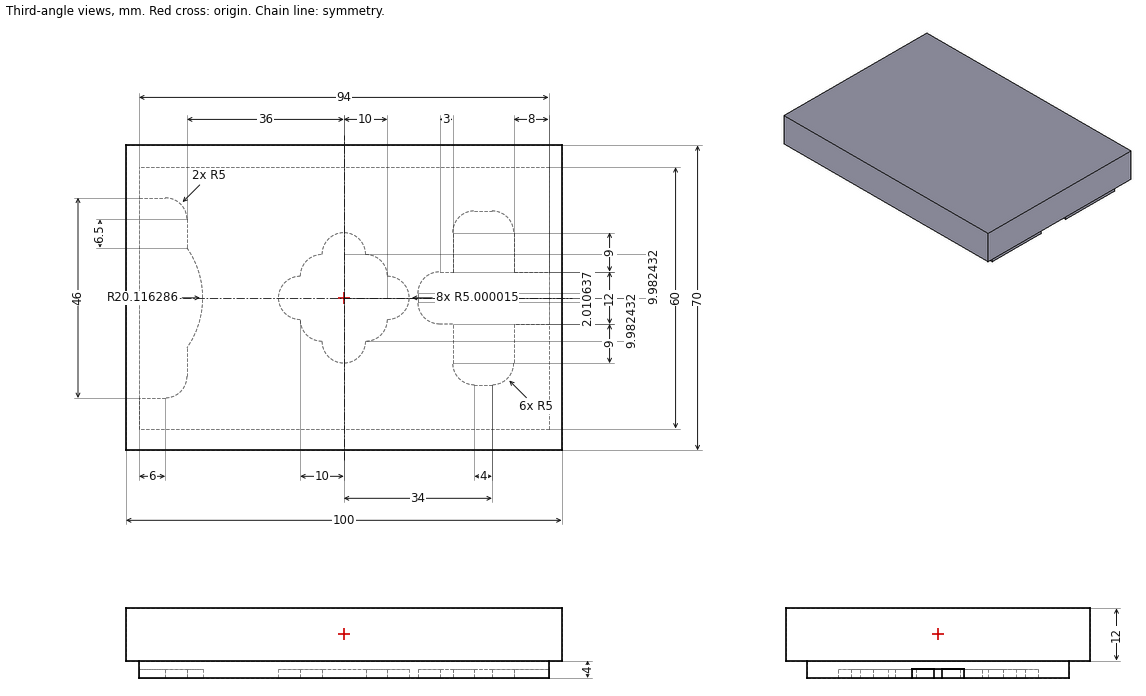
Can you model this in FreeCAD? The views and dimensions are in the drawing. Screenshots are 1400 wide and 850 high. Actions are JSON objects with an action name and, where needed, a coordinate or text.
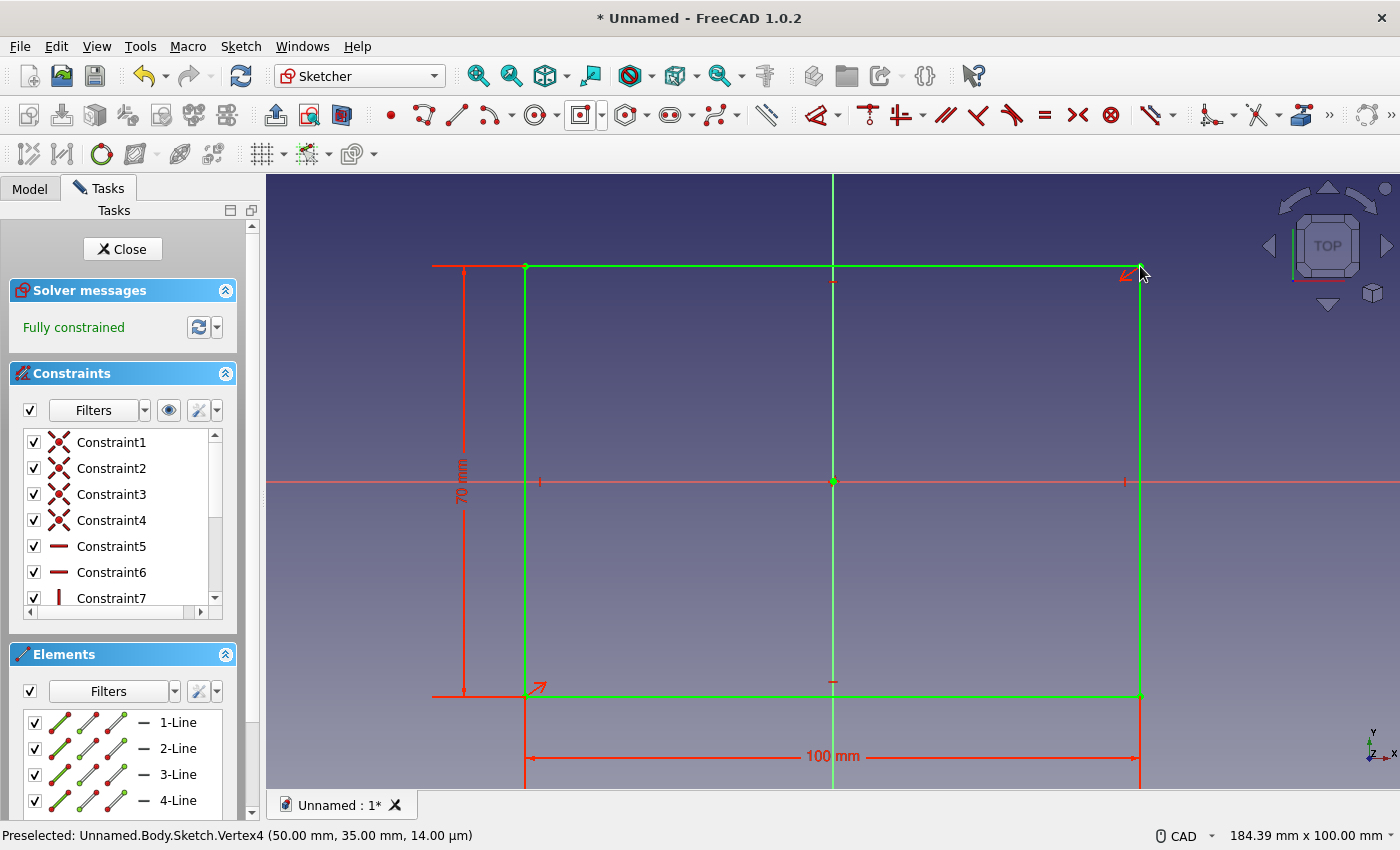
{"action": "left_click", "coordinate": [123, 249]}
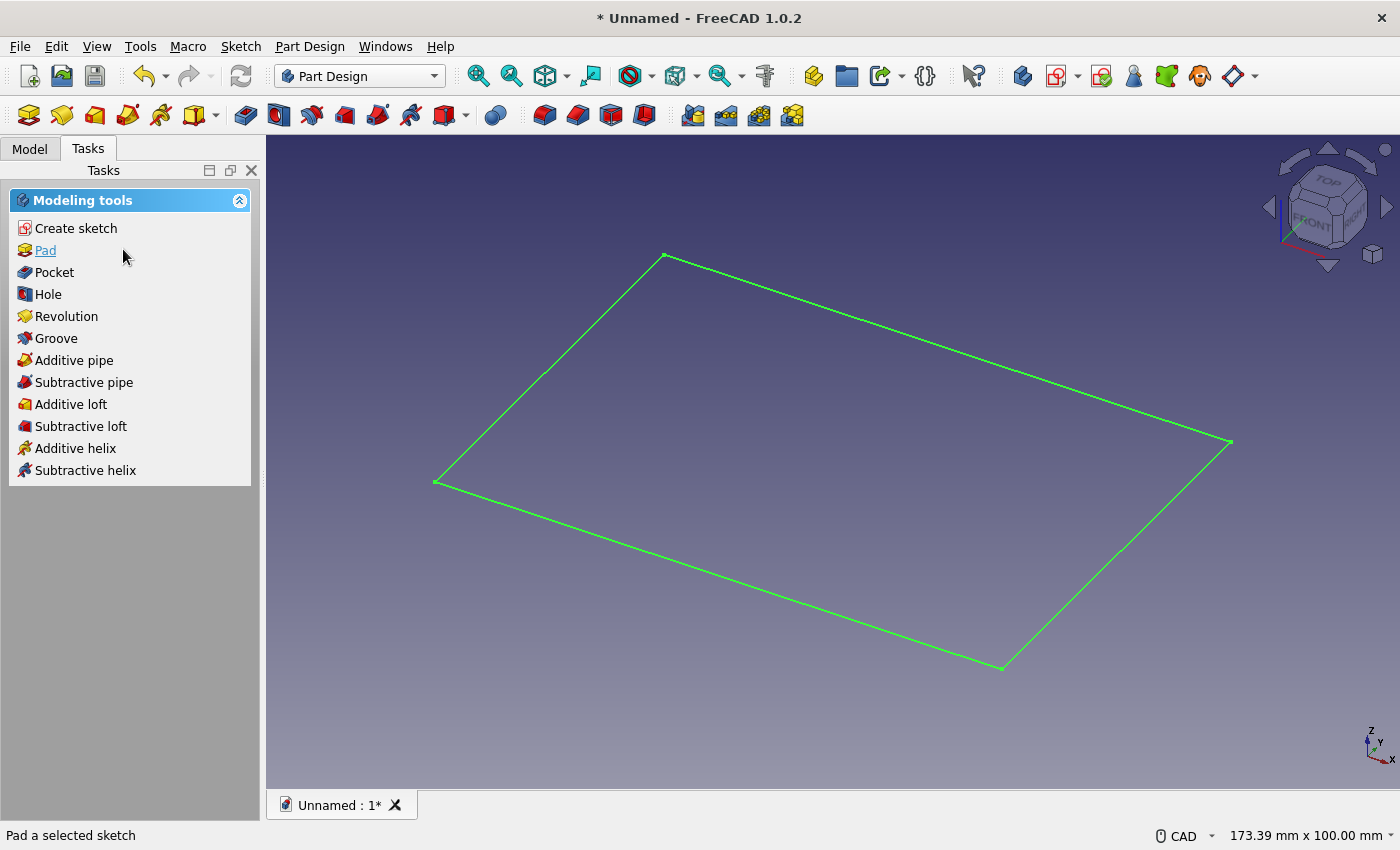
{"action": "left_click", "coordinate": [29, 116]}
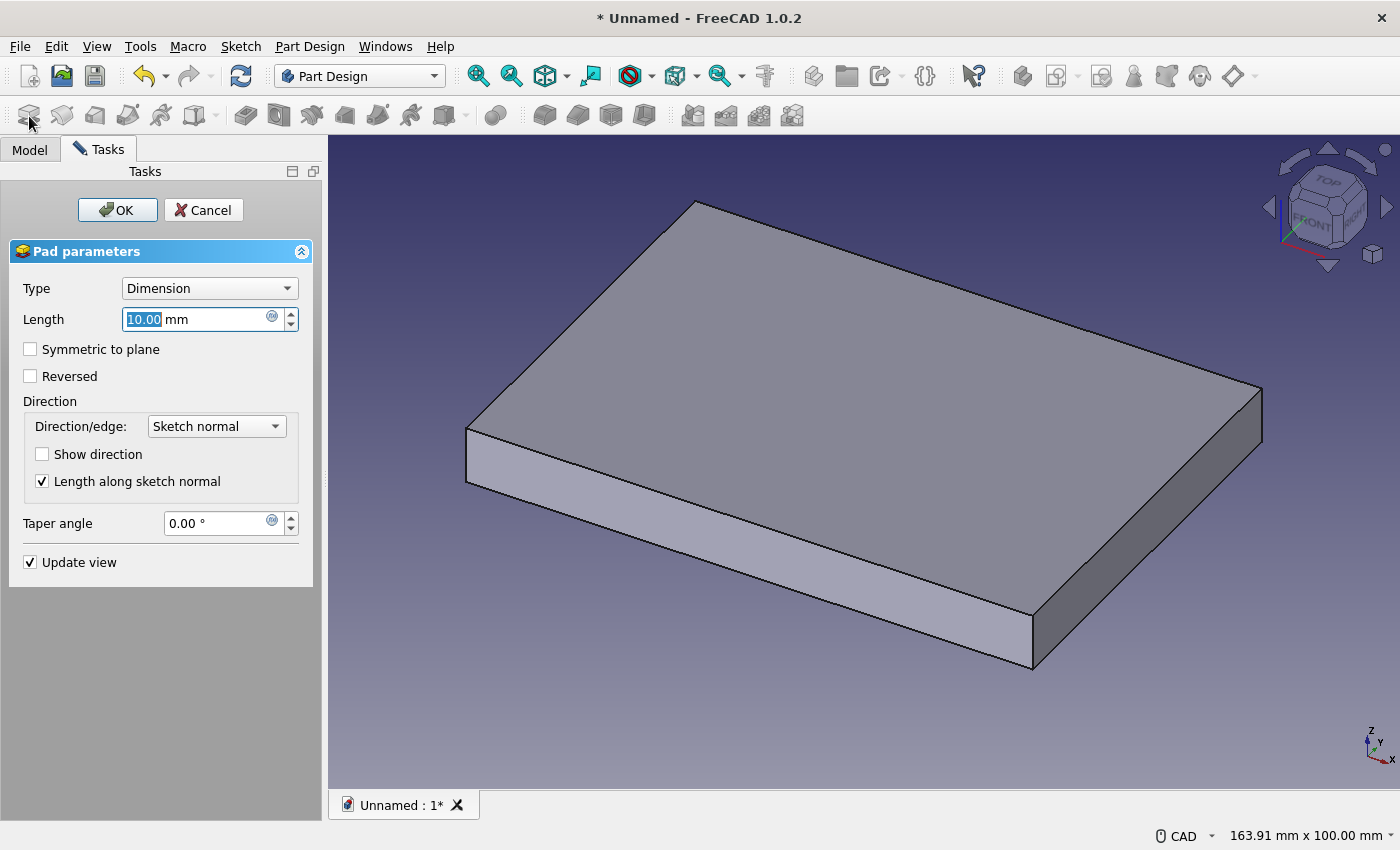
{"action": "type", "text": "12"}
{"action": "key", "text": "Tab"}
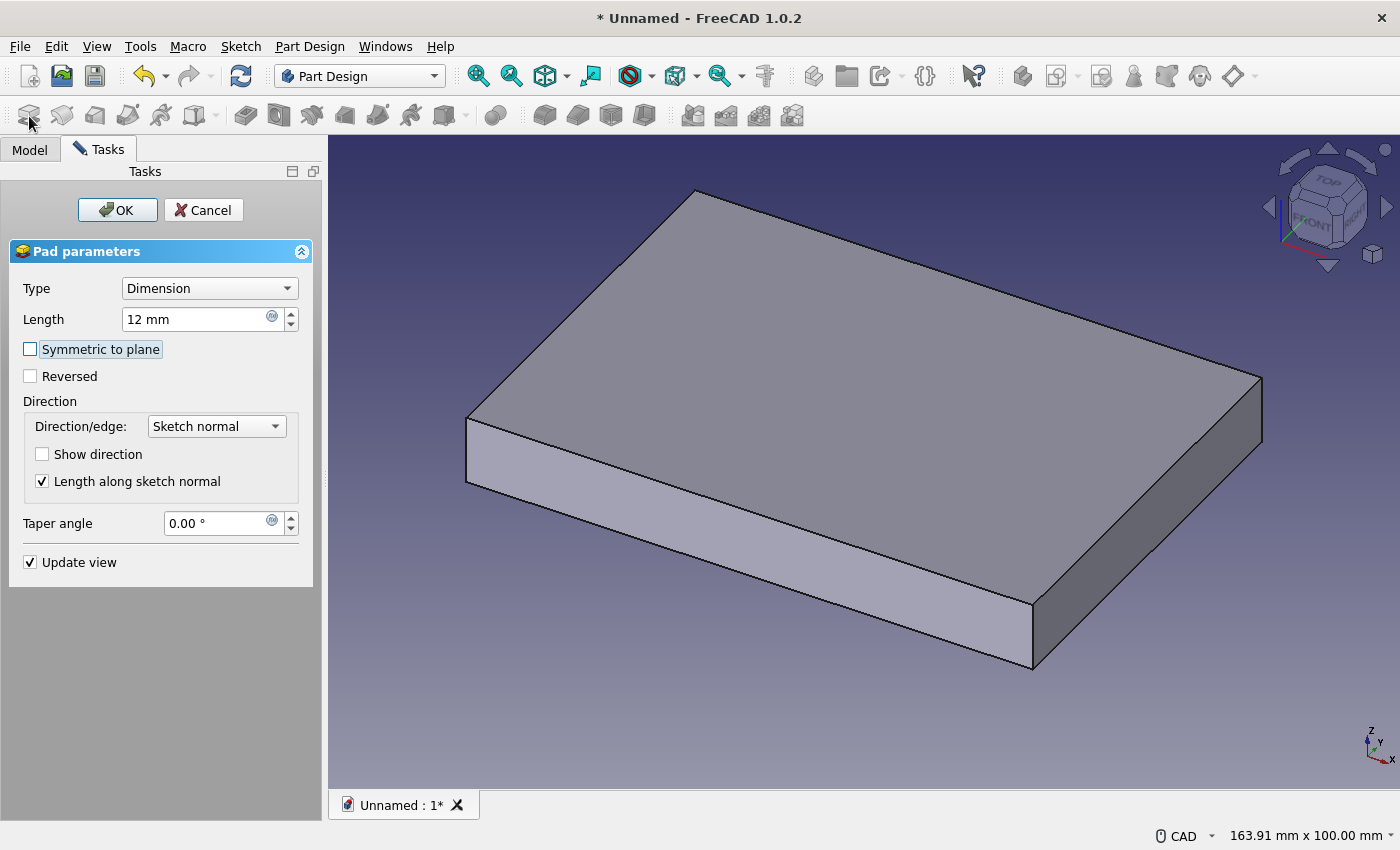
{"action": "left_click", "coordinate": [31, 349]}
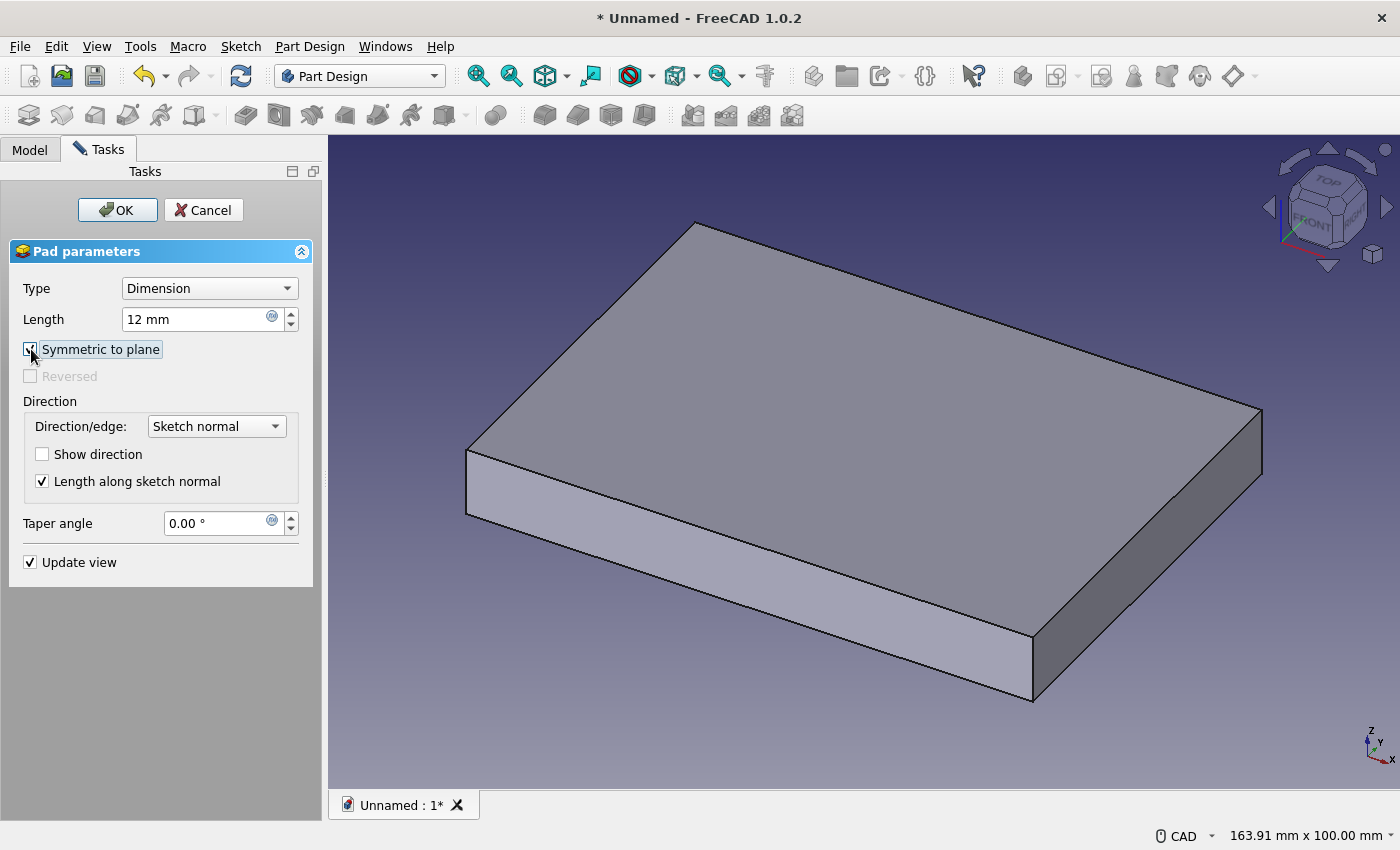
{"action": "left_click", "coordinate": [118, 210]}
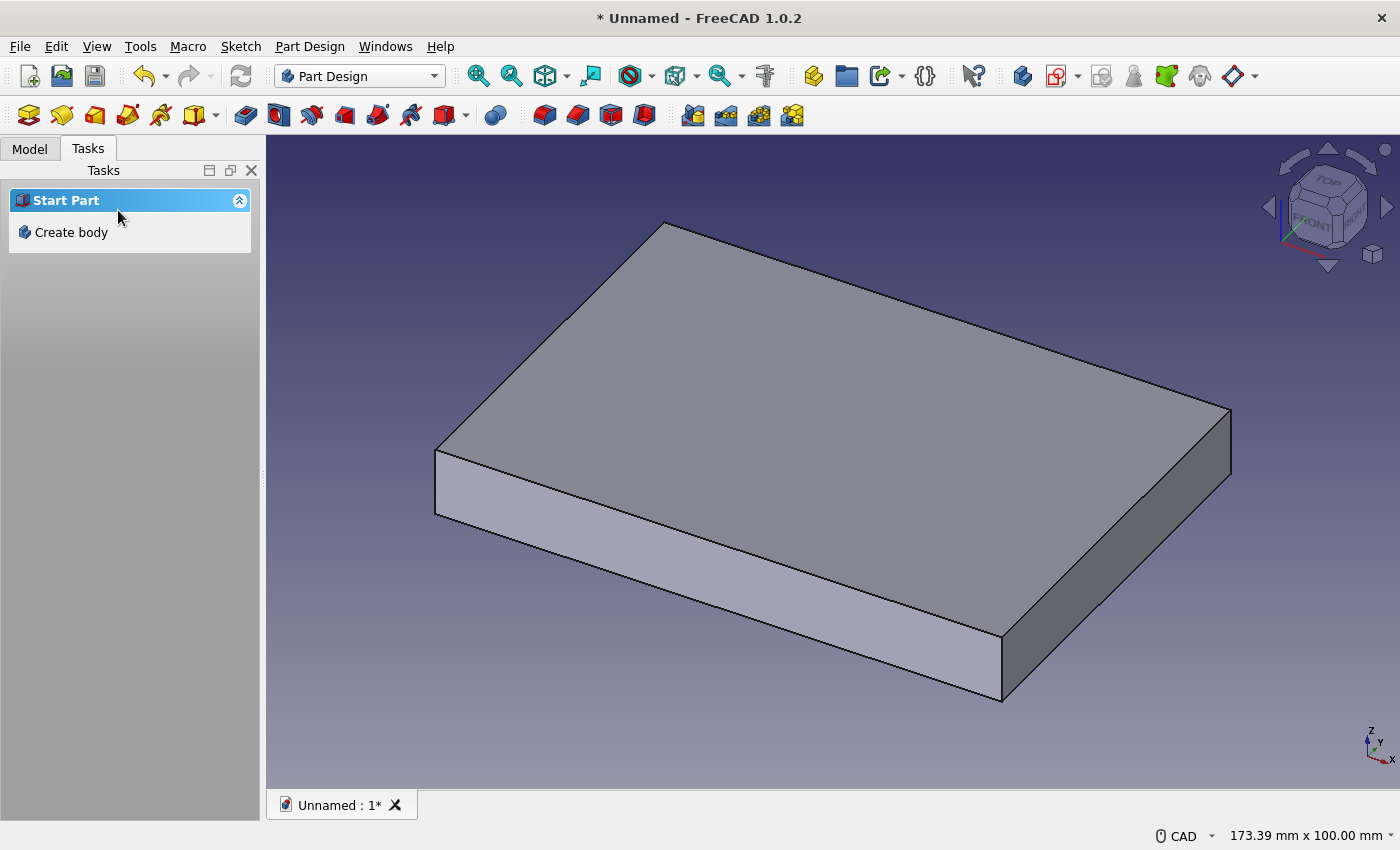
{"action": "key", "text": "5"}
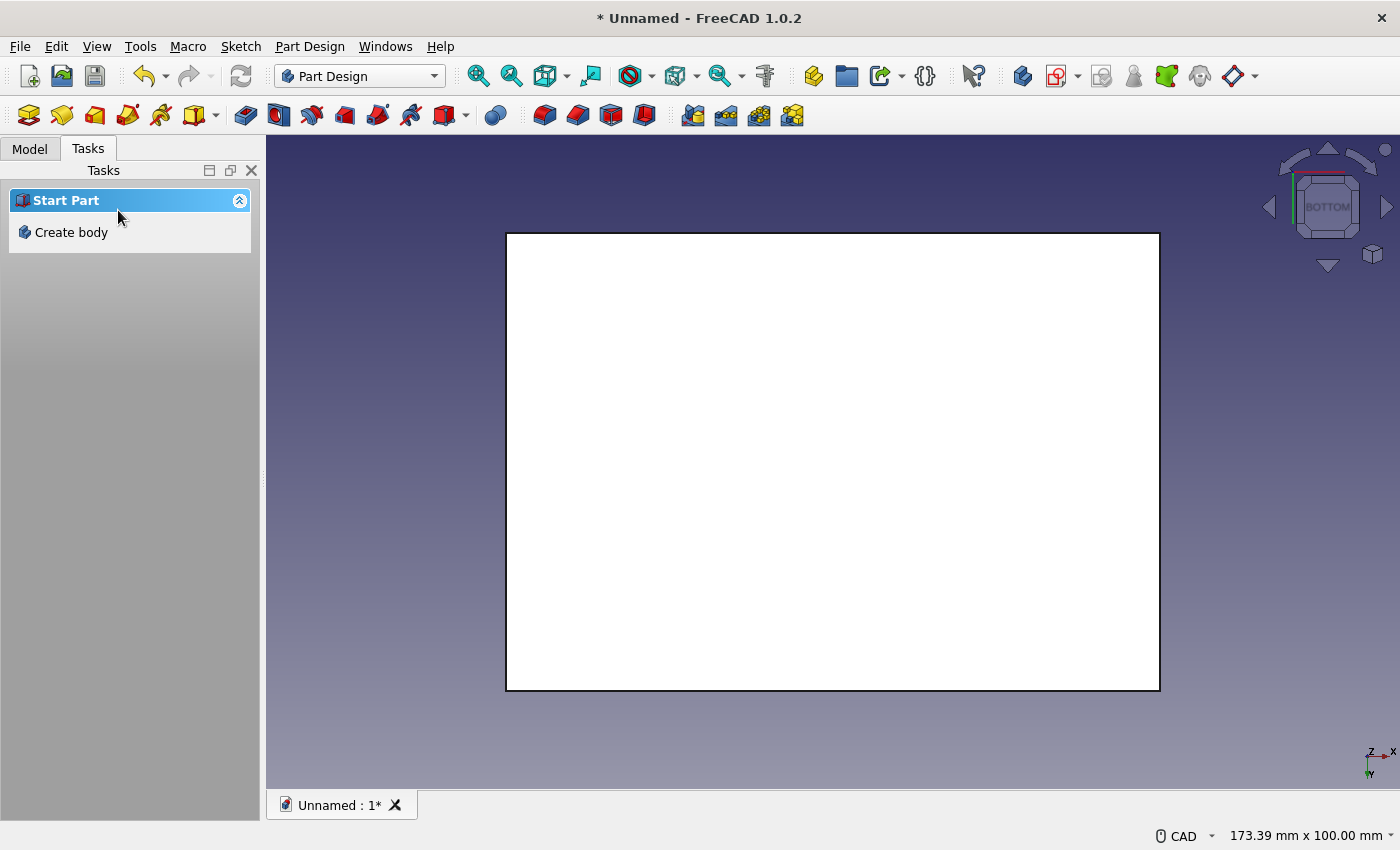
{"action": "left_click", "coordinate": [926, 461]}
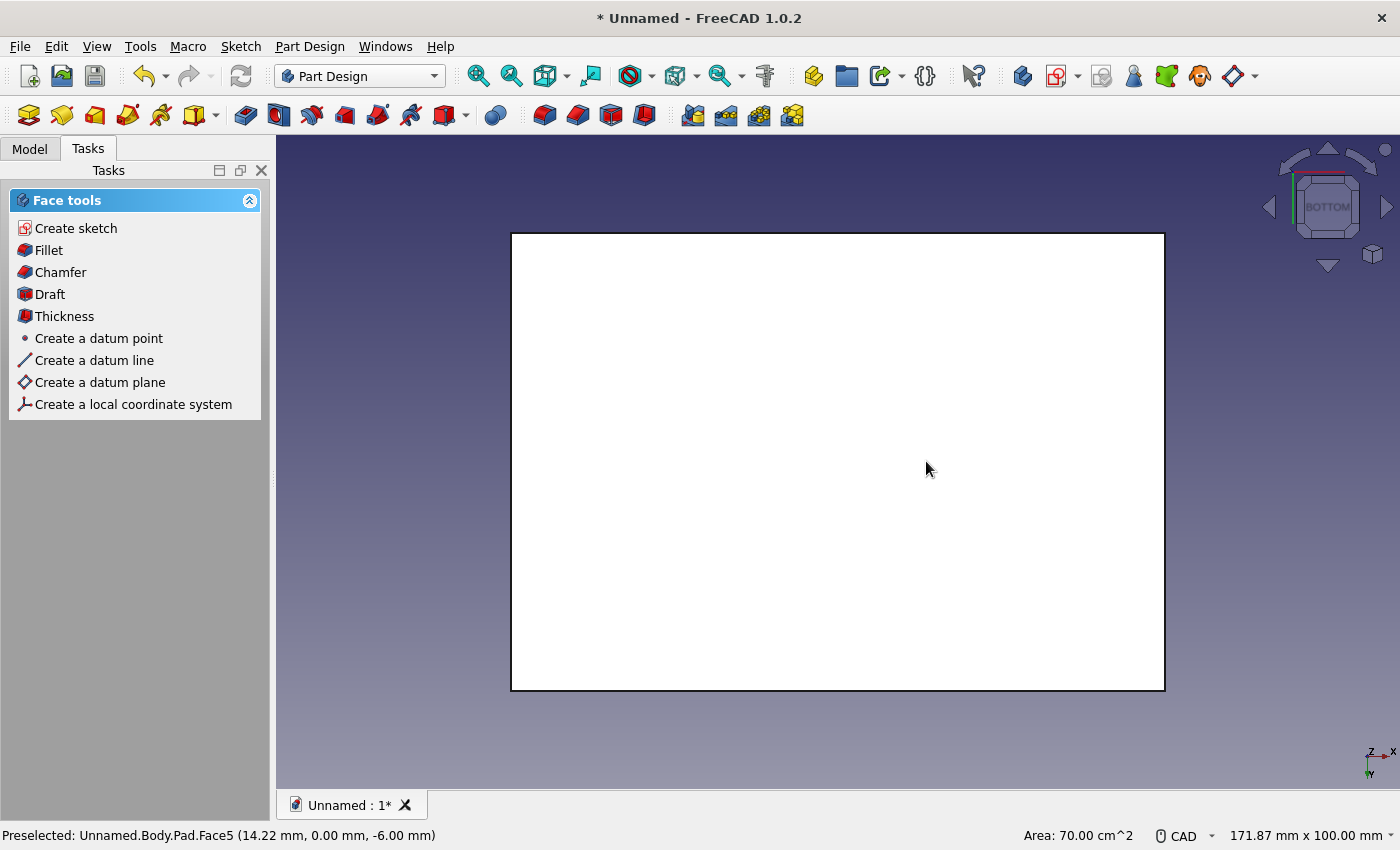
{"action": "left_click", "coordinate": [1056, 76]}